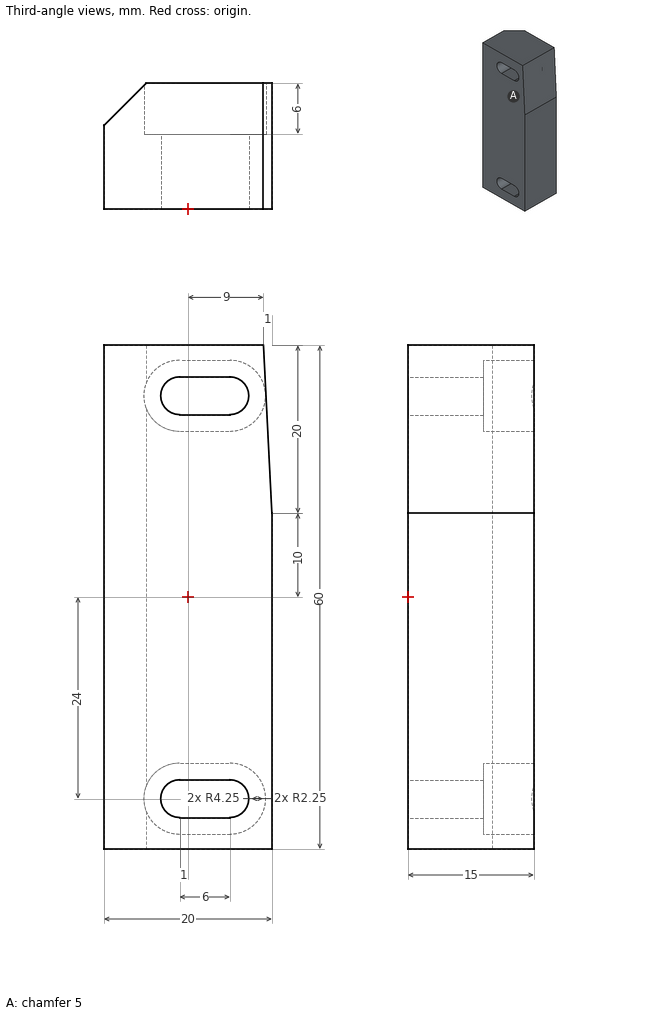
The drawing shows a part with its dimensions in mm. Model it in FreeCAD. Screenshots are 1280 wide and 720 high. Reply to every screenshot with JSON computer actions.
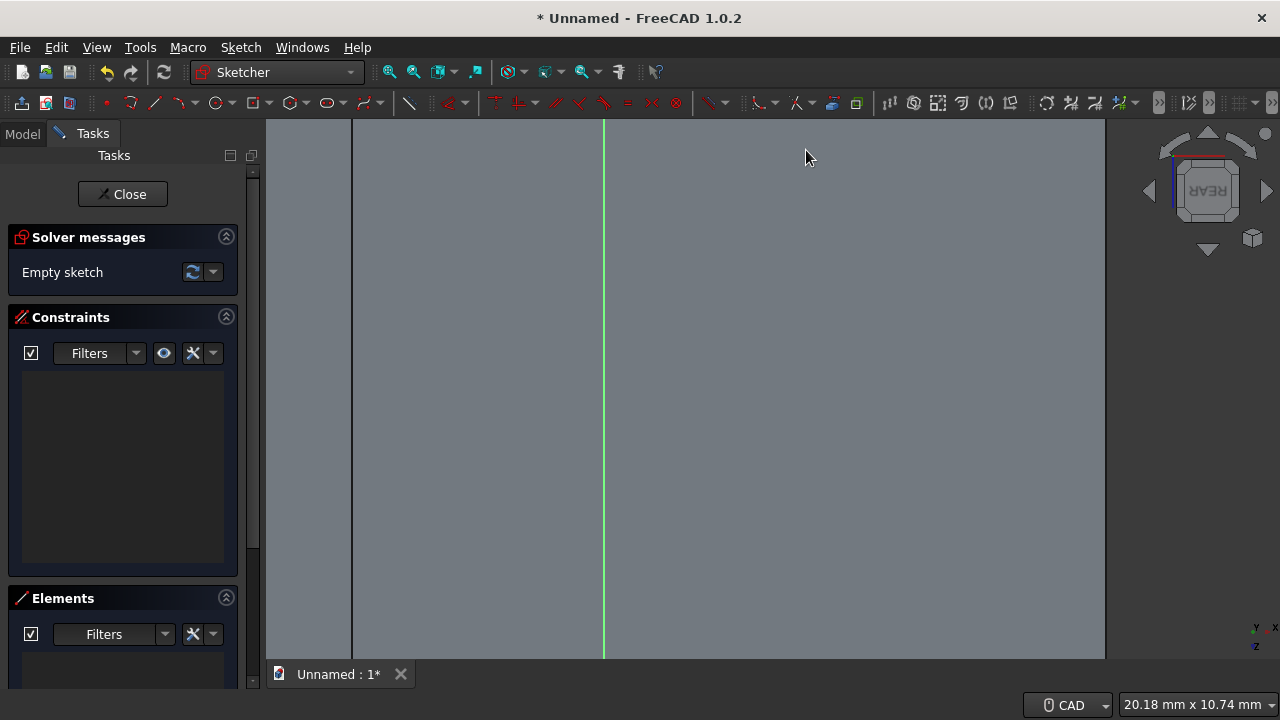
{"action": "left_click", "coordinate": [328, 104]}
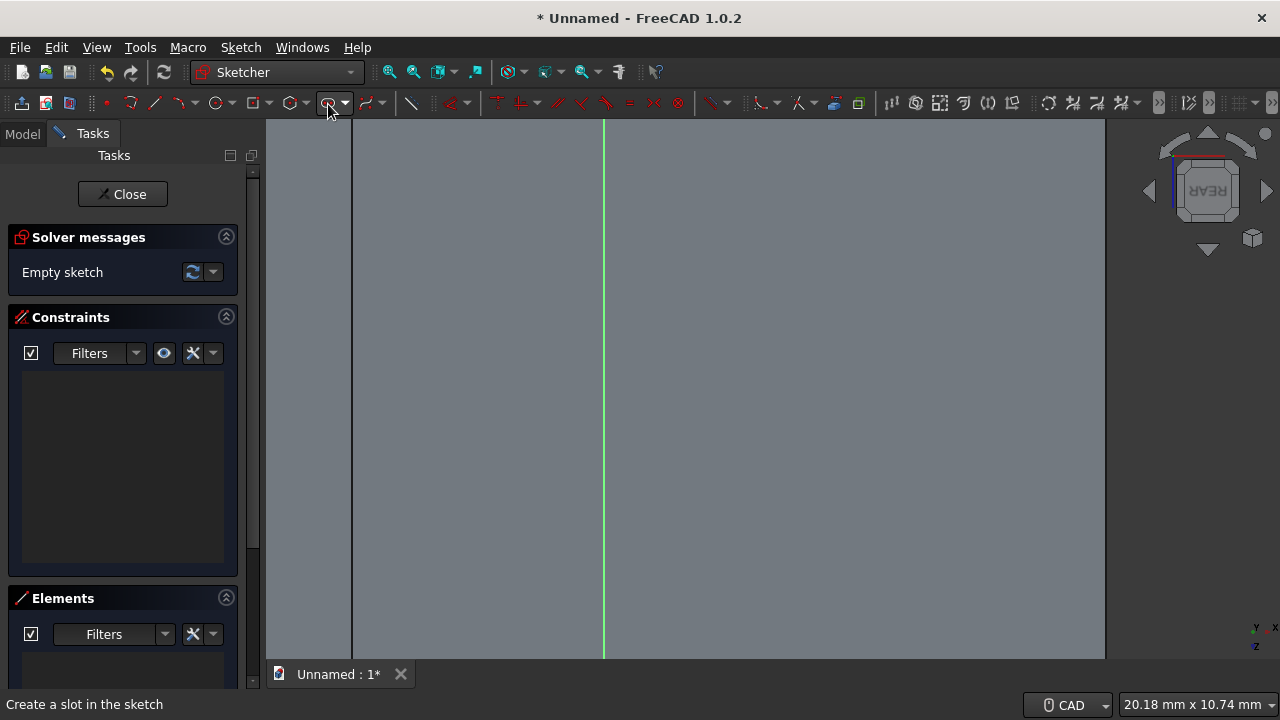
{"action": "left_click", "coordinate": [553, 389]}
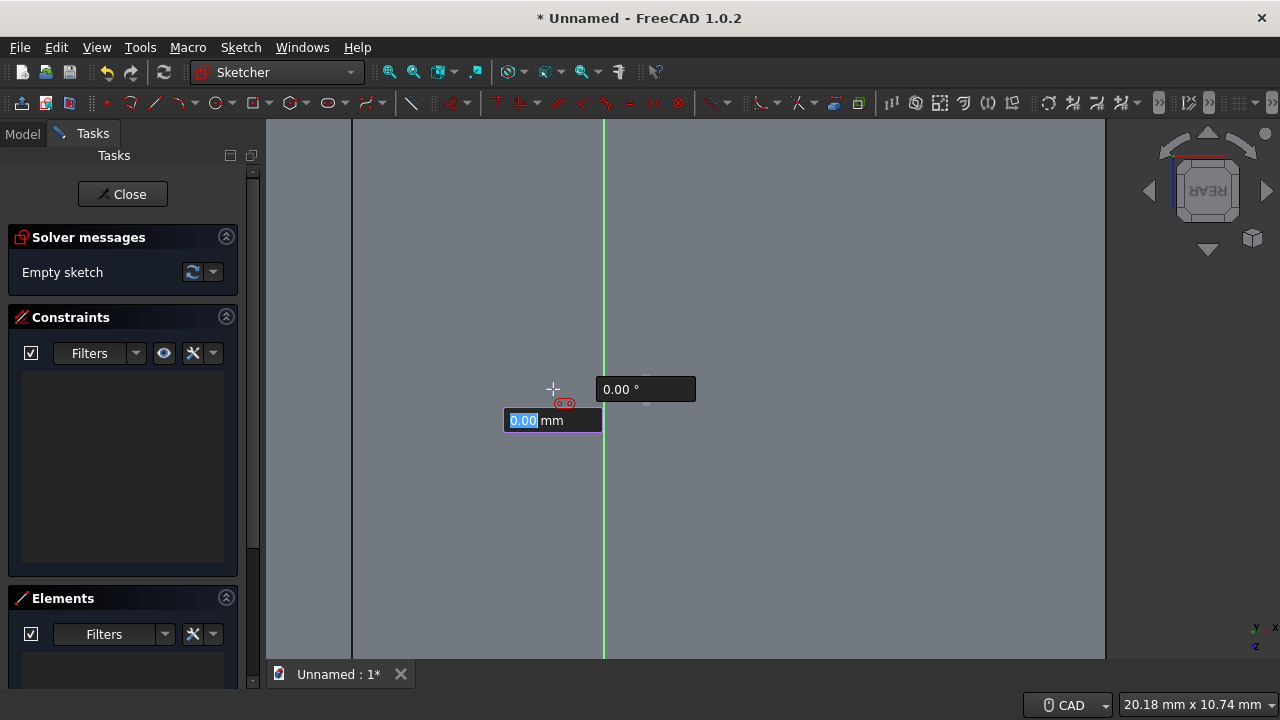
{"action": "left_click", "coordinate": [855, 389]}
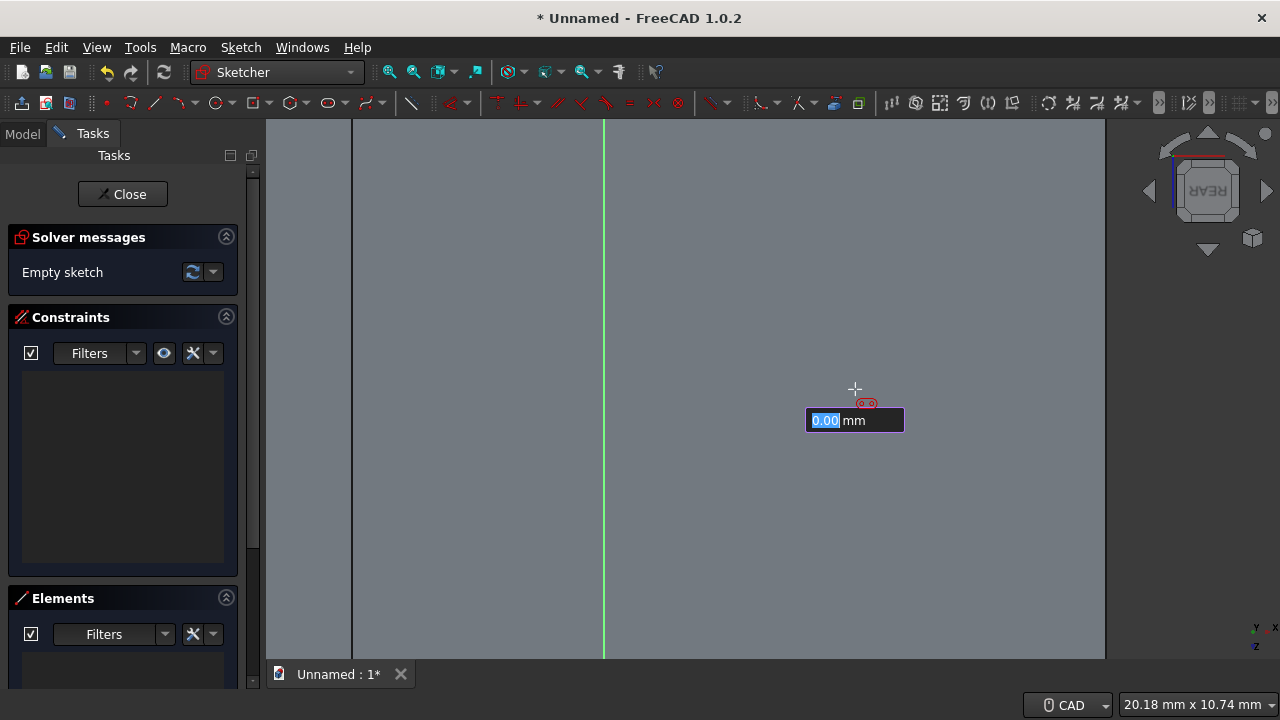
{"action": "left_click", "coordinate": [704, 502]}
{"action": "key", "text": "Escape"}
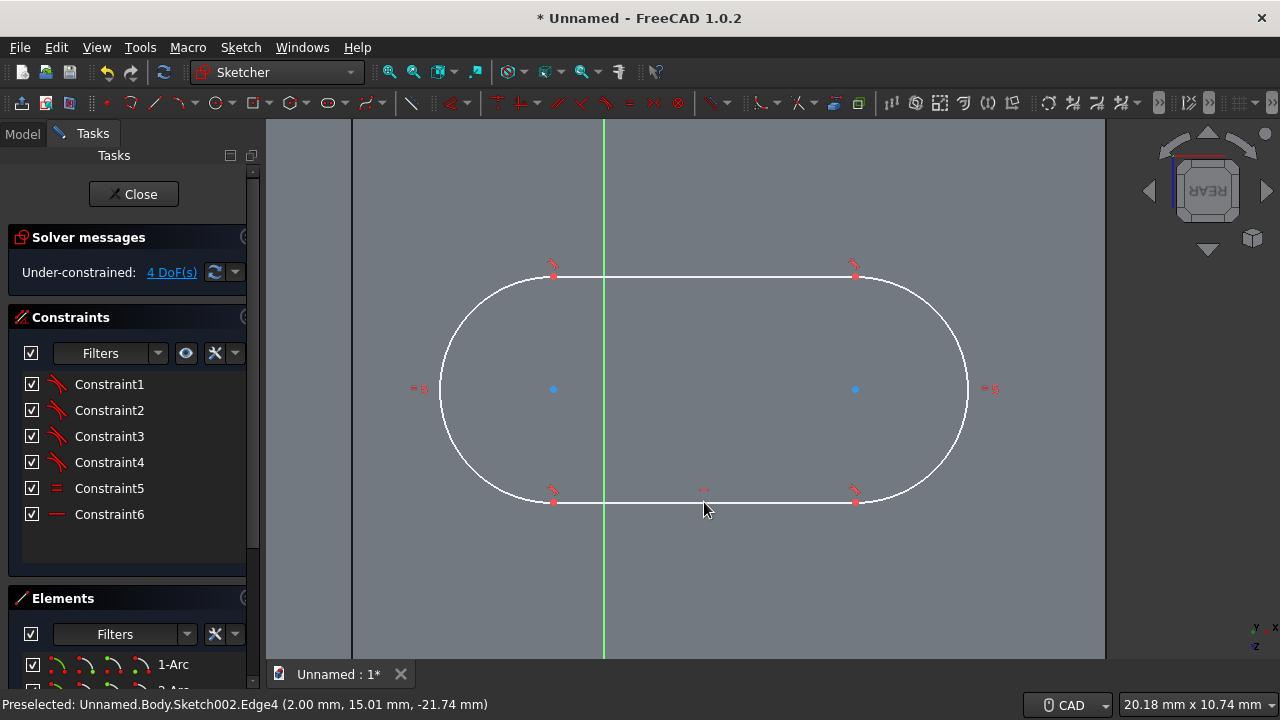
{"action": "left_click", "coordinate": [450, 104]}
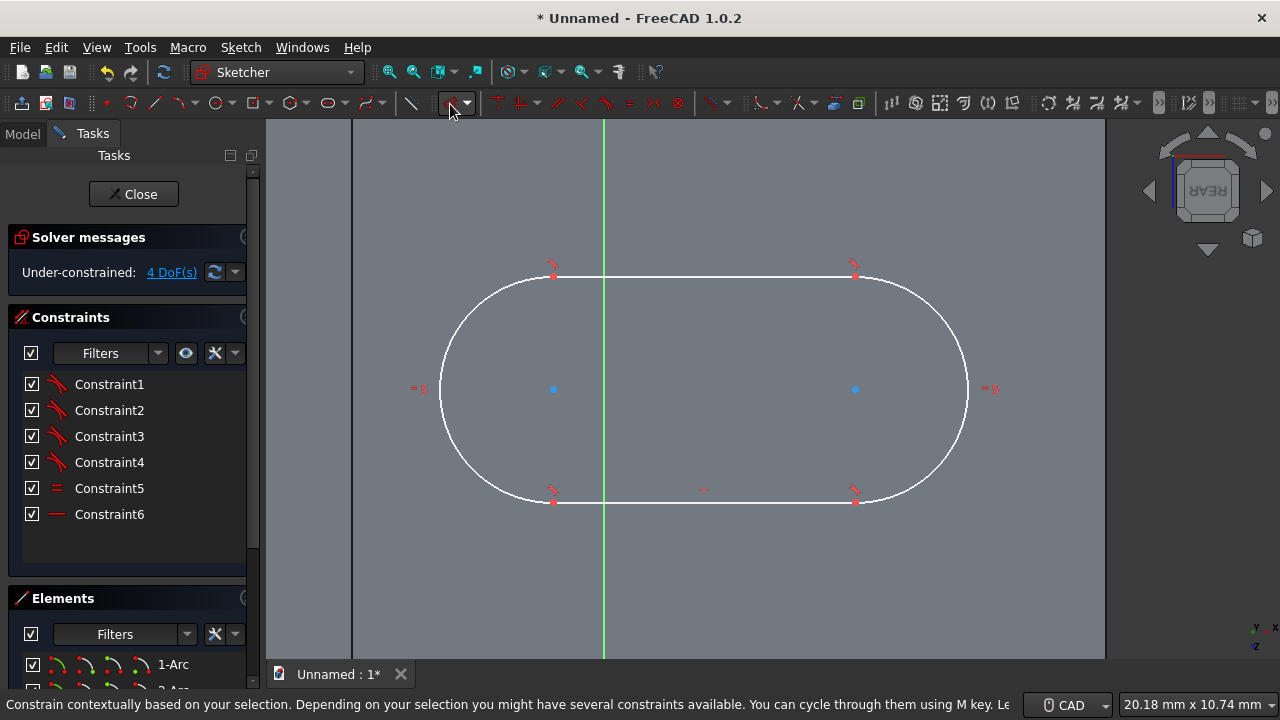
{"action": "left_click", "coordinate": [462, 324]}
{"action": "left_click", "coordinate": [436, 305]}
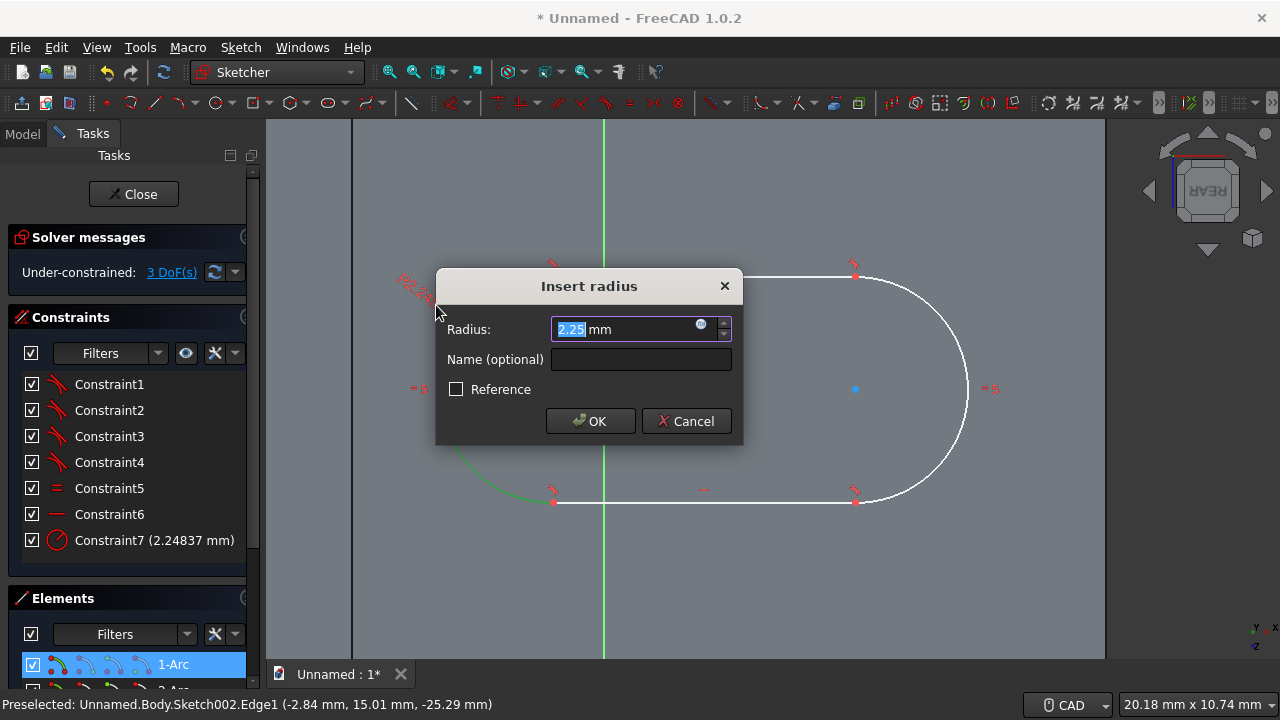
{"action": "type", "text": "2.25"}
{"action": "key", "text": "Return"}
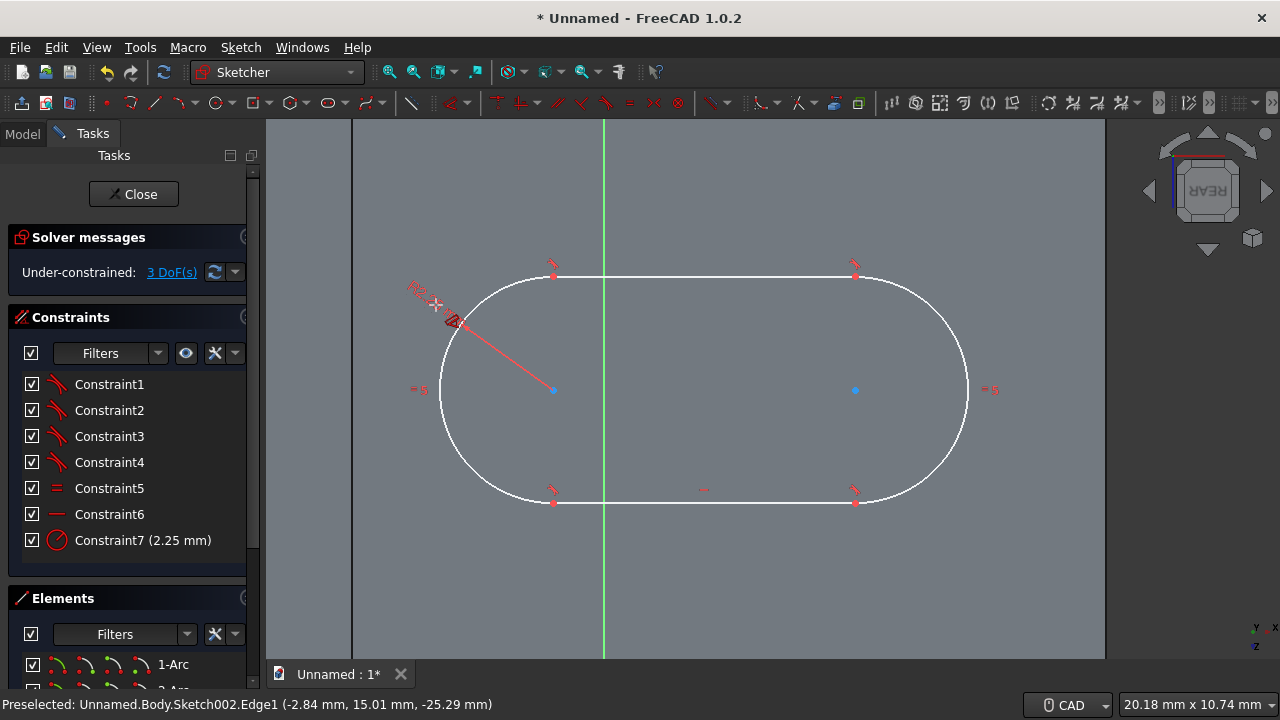
{"action": "left_click", "coordinate": [644, 277]}
{"action": "left_click", "coordinate": [704, 243]}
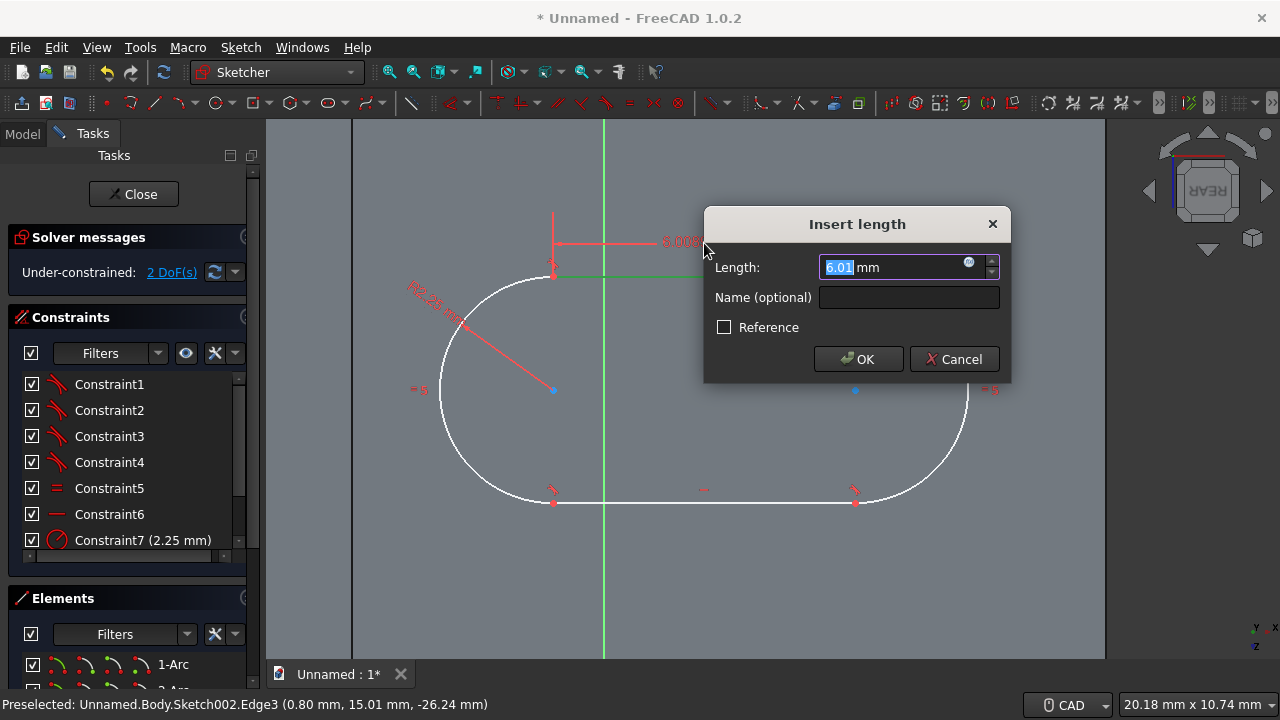
{"action": "type", "text": "6"}
{"action": "key", "text": "Return"}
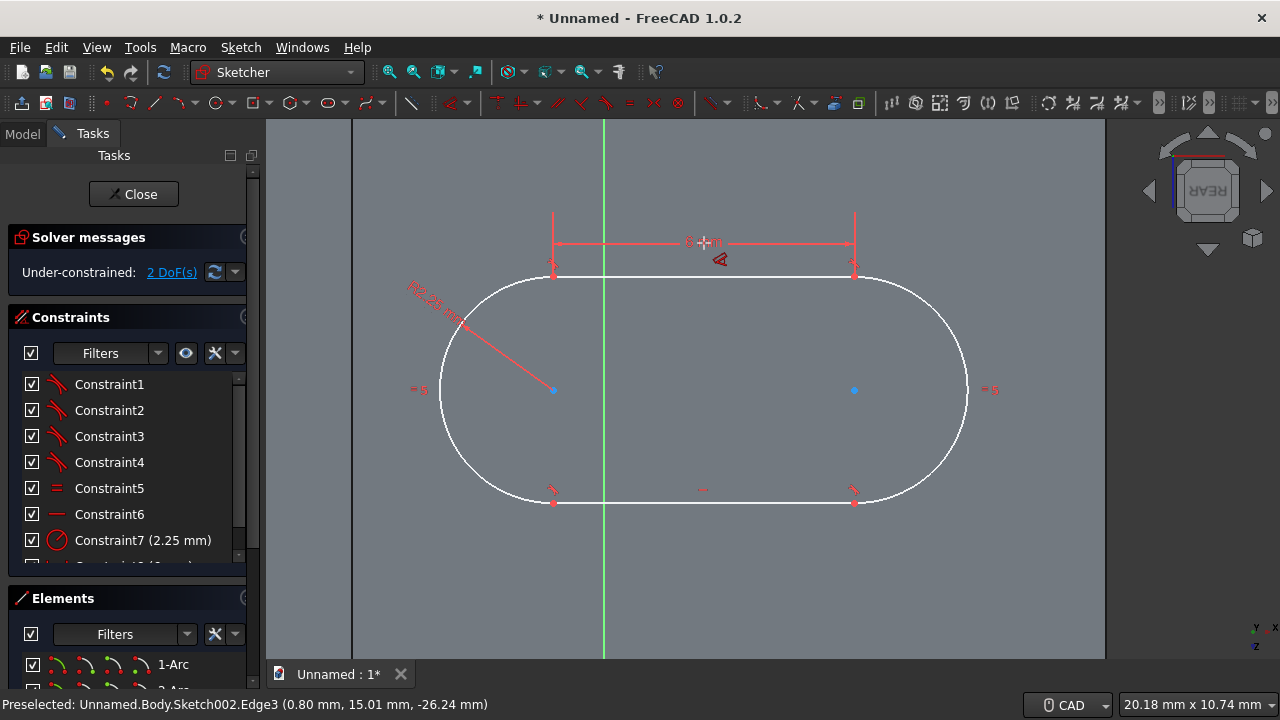
{"action": "left_click", "coordinate": [553, 277]}
{"action": "left_click", "coordinate": [578, 243]}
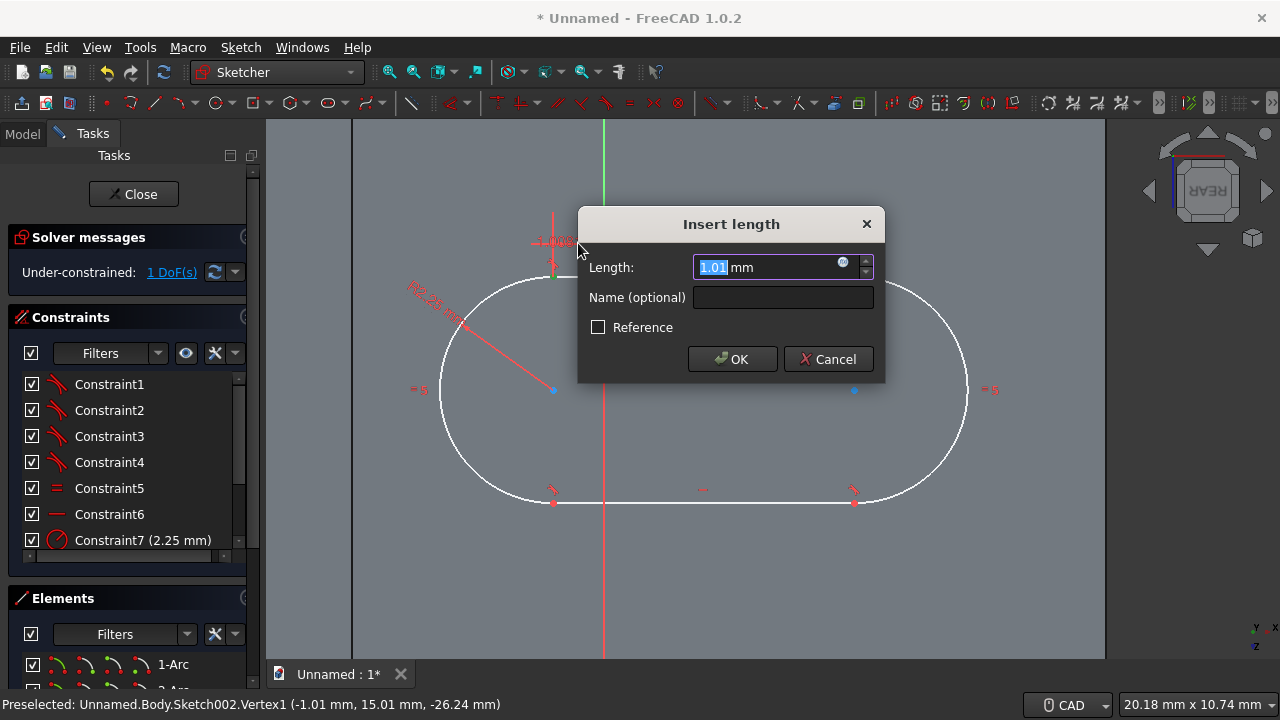
{"action": "type", "text": "1"}
{"action": "key", "text": "Return"}